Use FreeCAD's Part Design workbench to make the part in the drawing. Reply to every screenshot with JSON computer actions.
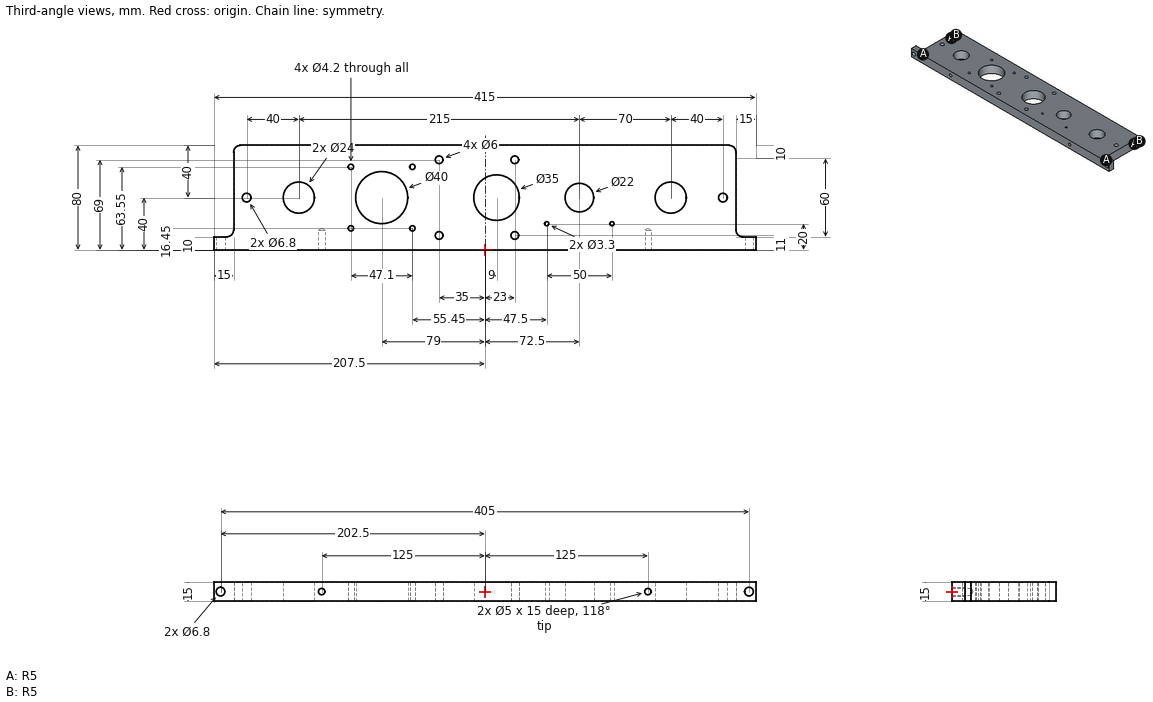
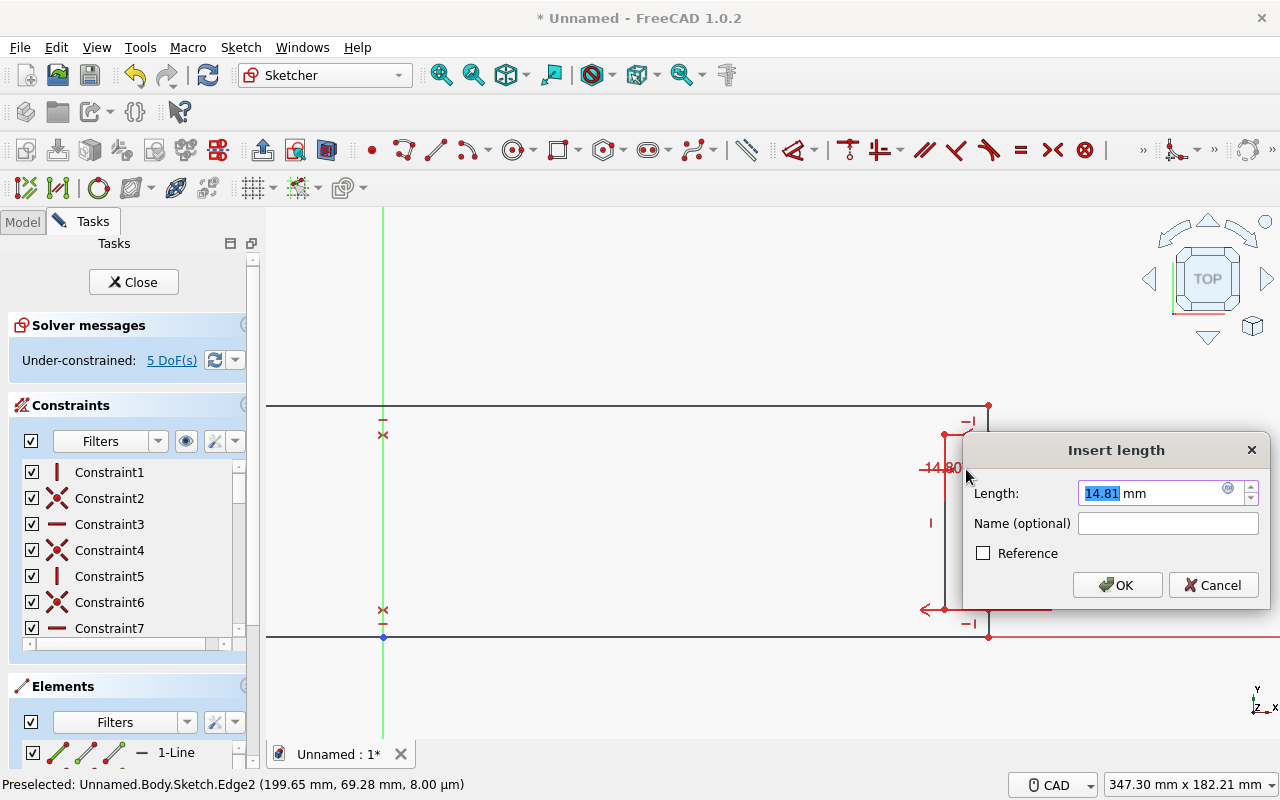
{"action": "type", "text": "15"}
{"action": "key", "text": "Return"}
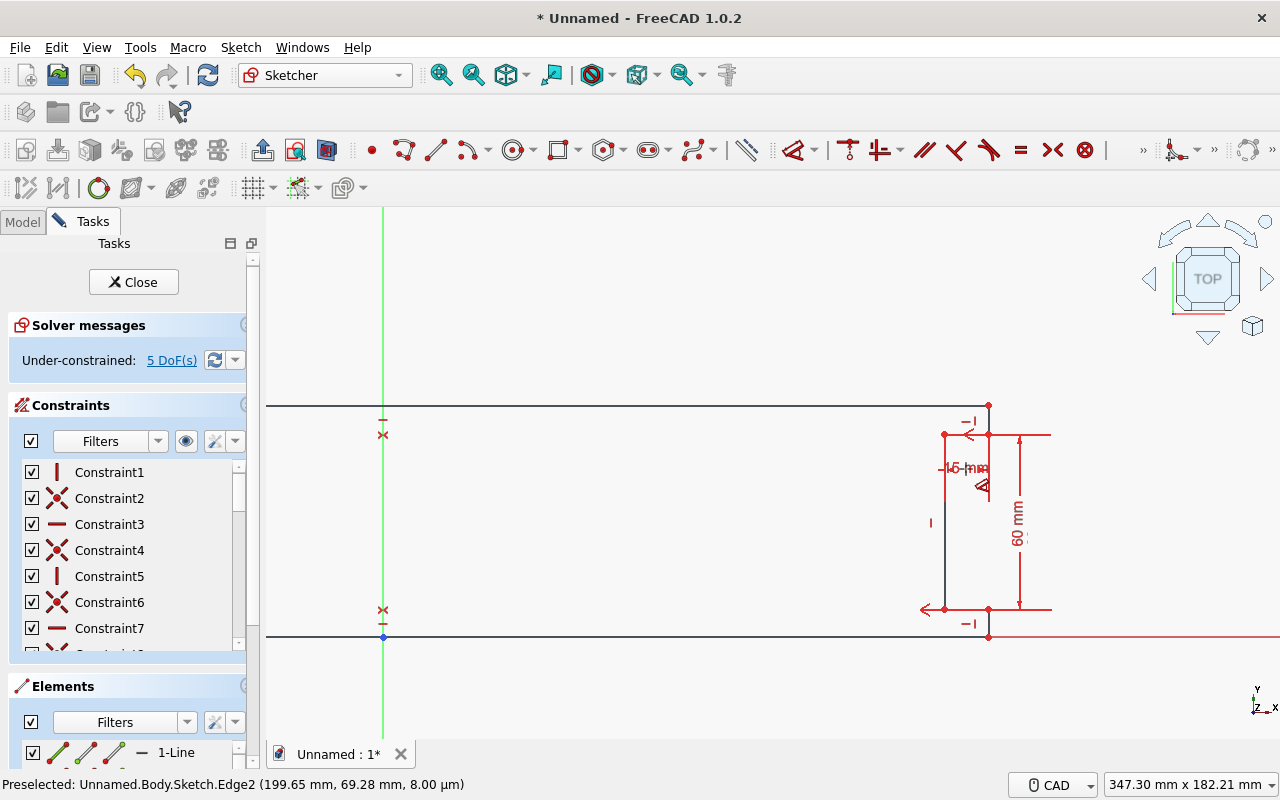
{"action": "scroll", "coordinate": [989, 423], "scroll_direction": "up", "scroll_amount": 2}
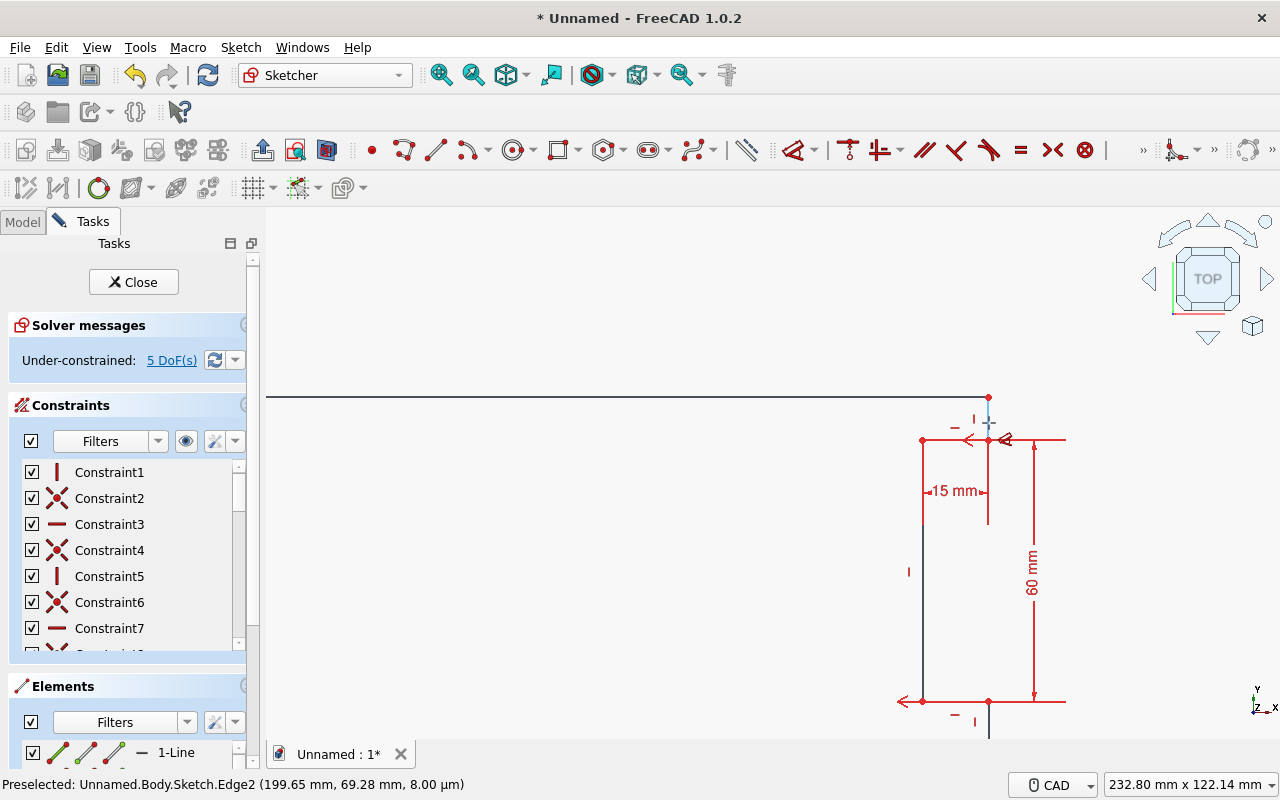
{"action": "left_click", "coordinate": [988, 423]}
{"action": "left_click", "coordinate": [1022, 419]}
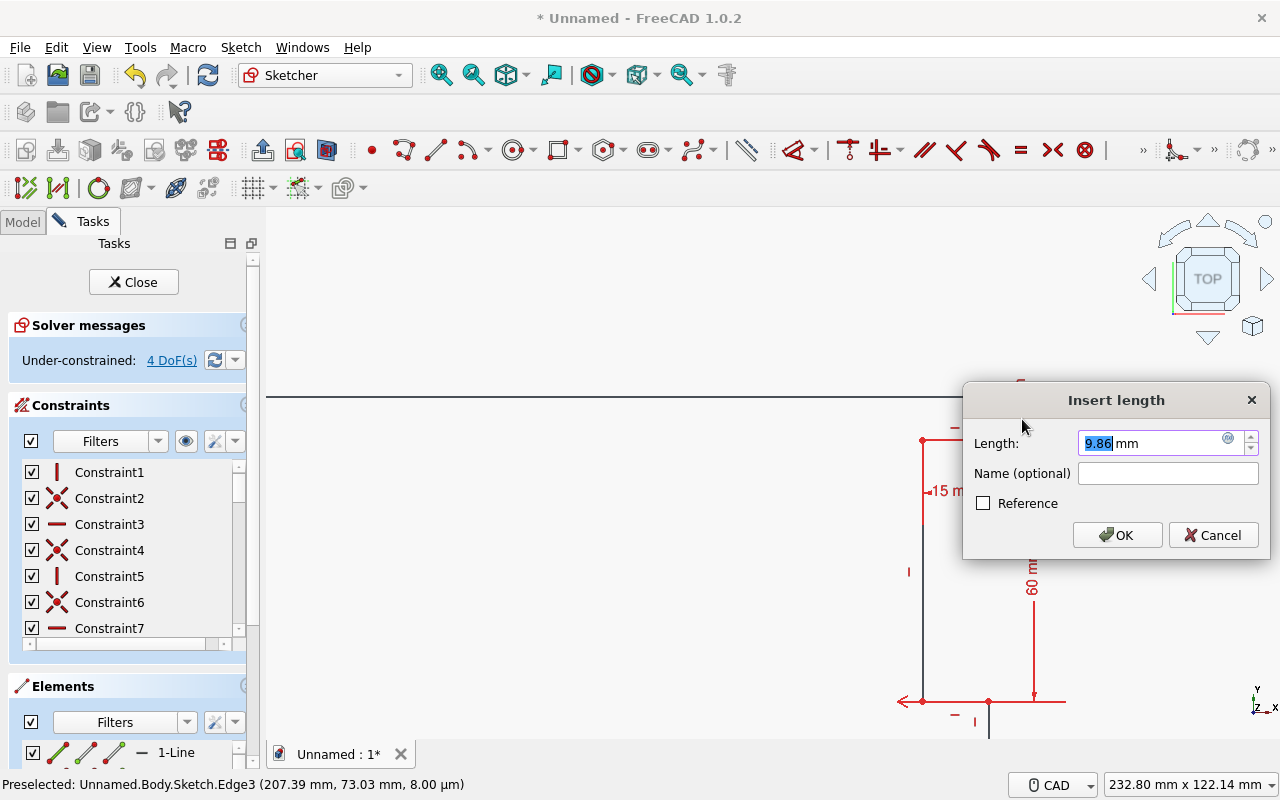
{"action": "type", "text": "10"}
{"action": "key", "text": "Return"}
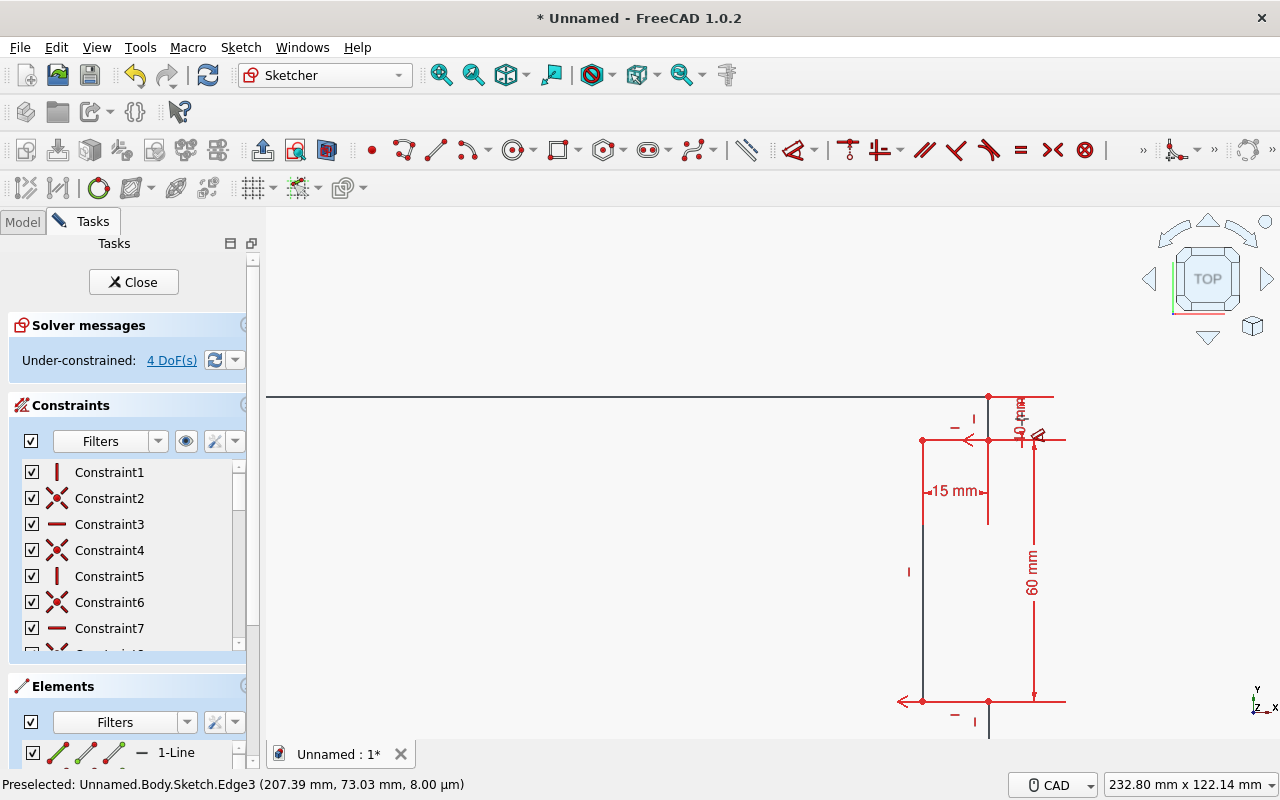
{"action": "scroll", "coordinate": [972, 432], "scroll_direction": "down", "scroll_amount": 6}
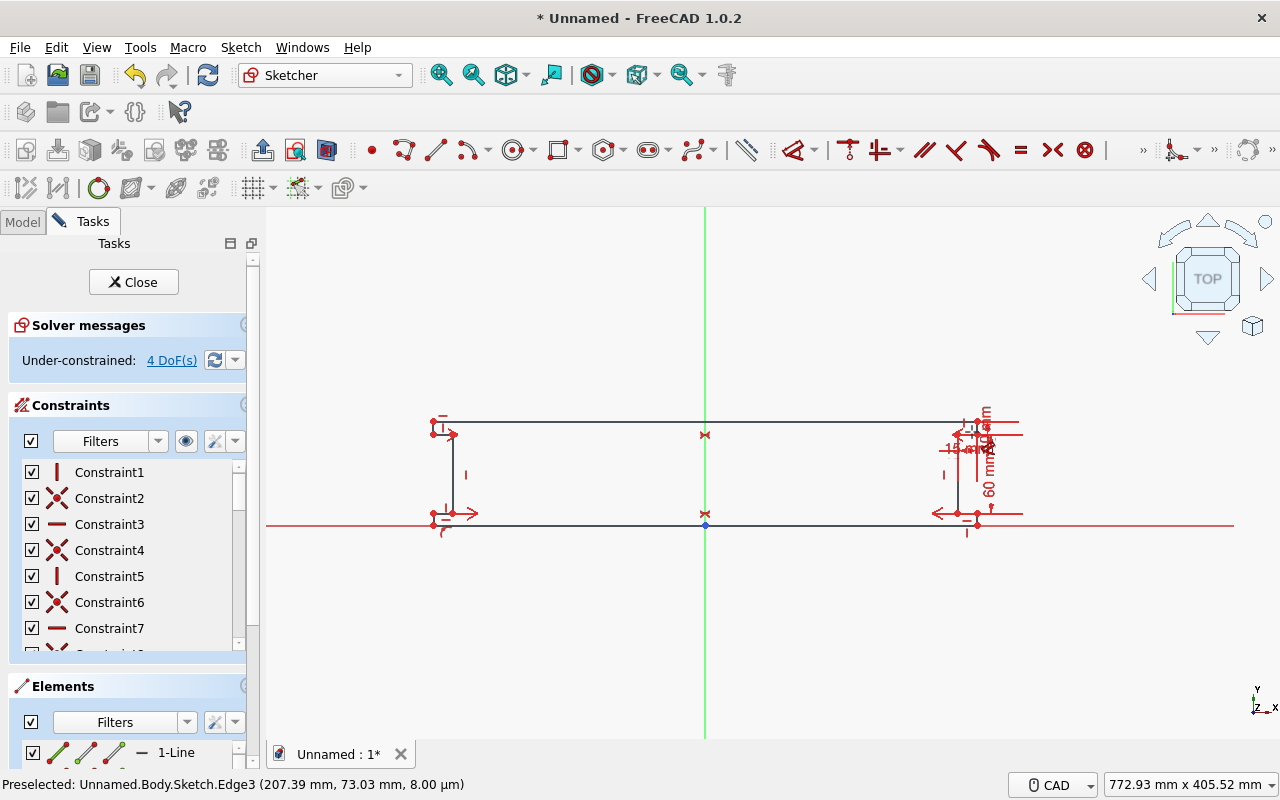
{"action": "scroll", "coordinate": [447, 514], "scroll_direction": "up", "scroll_amount": 5}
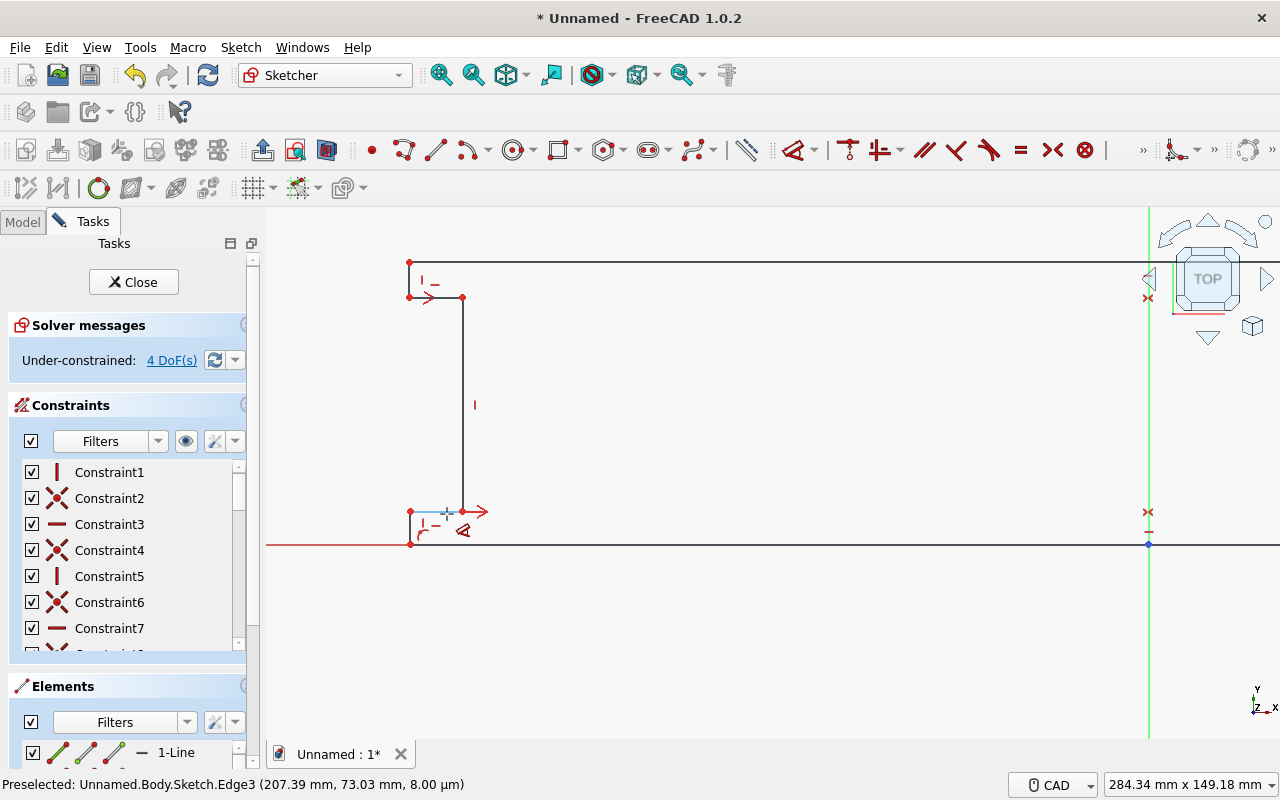
{"action": "left_click", "coordinate": [447, 512]}
{"action": "left_click", "coordinate": [436, 478]}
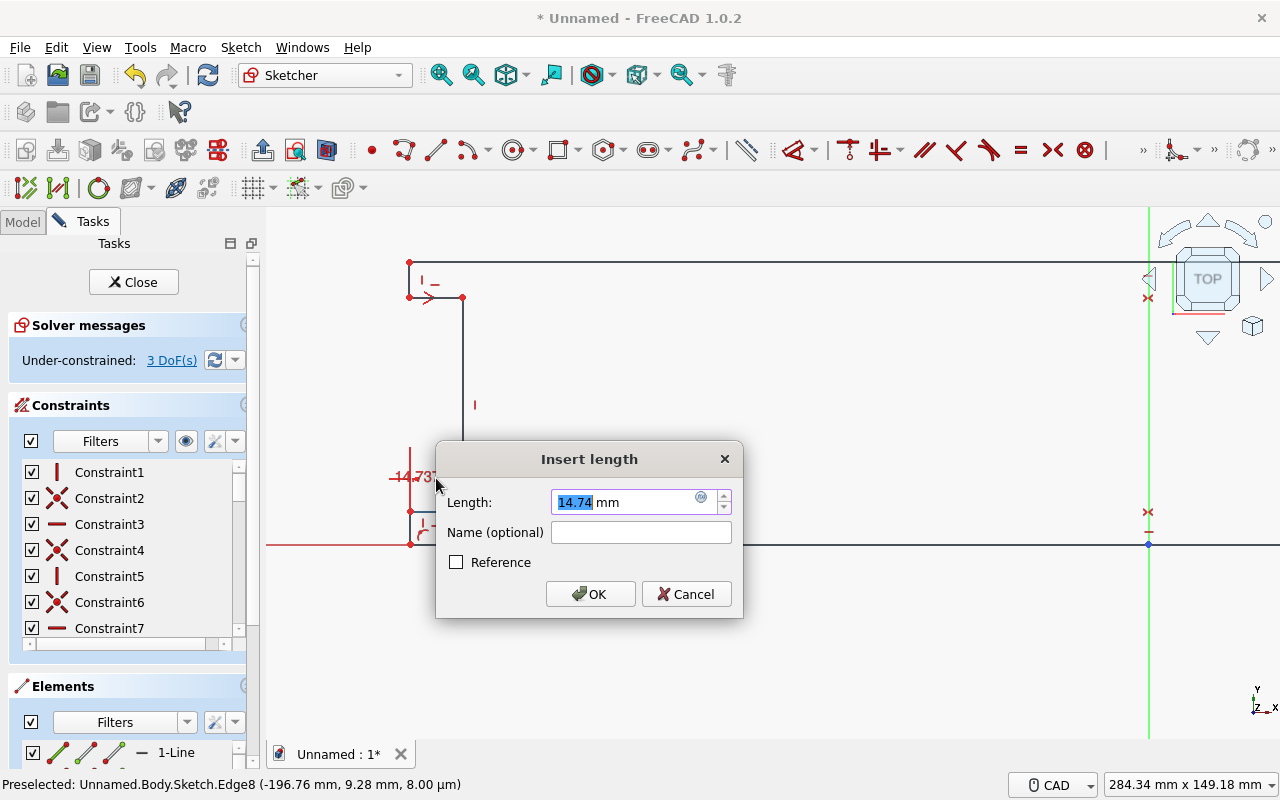
{"action": "type", "text": "15"}
{"action": "key", "text": "Return"}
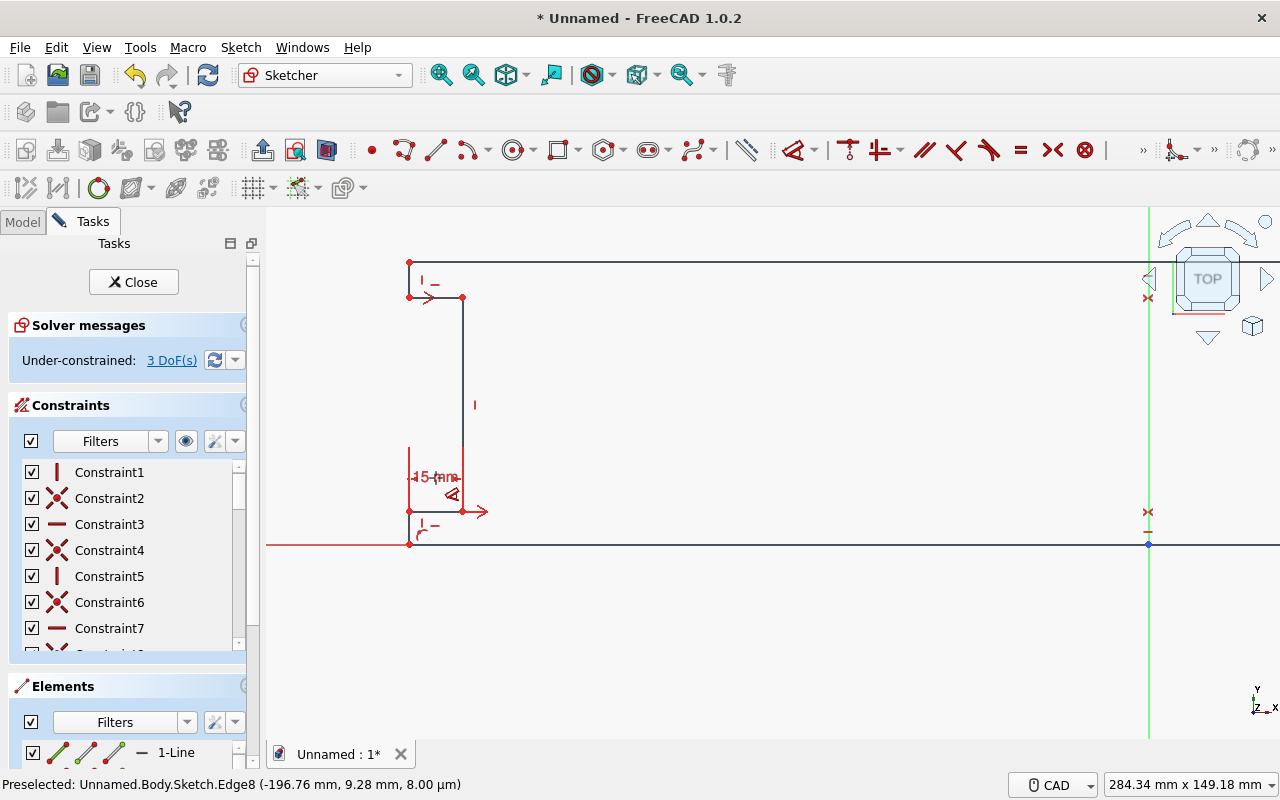
{"action": "scroll", "coordinate": [409, 522], "scroll_direction": "up", "scroll_amount": 2}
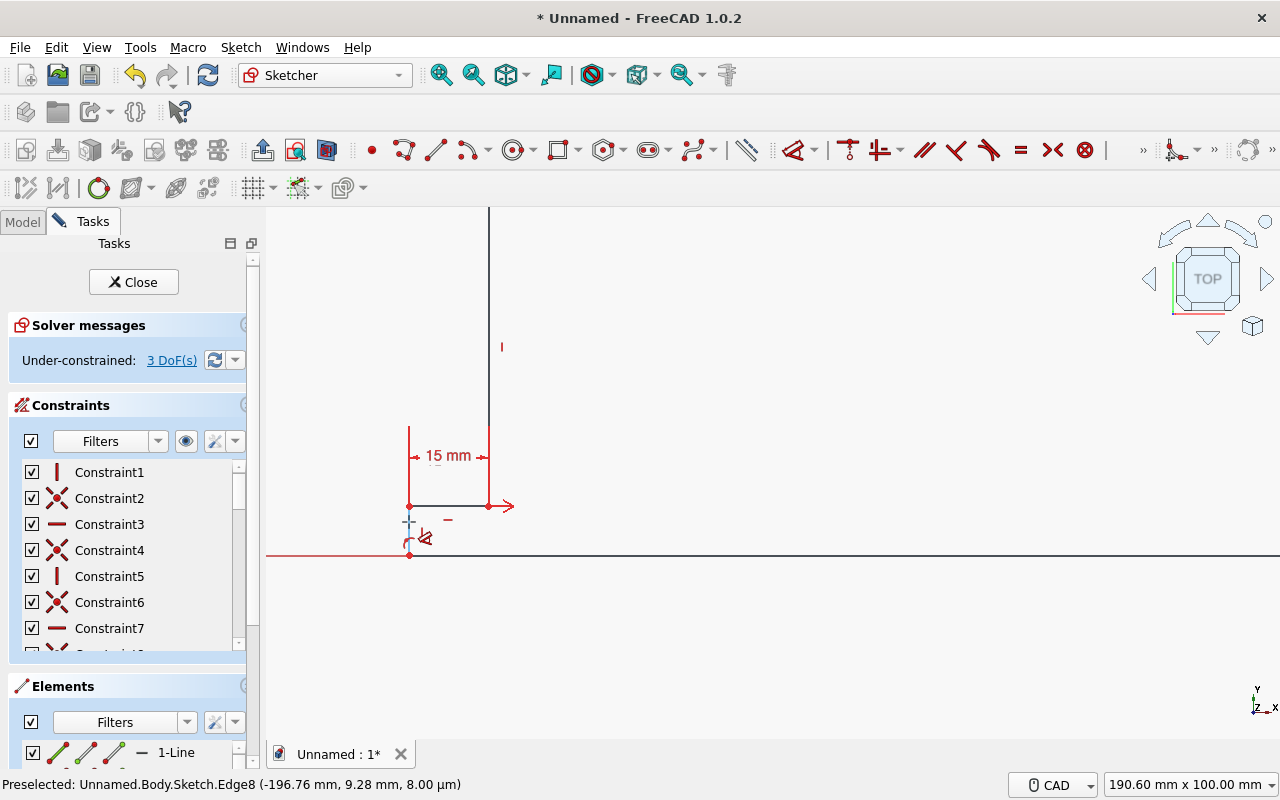
{"action": "left_click", "coordinate": [409, 521]}
{"action": "left_click", "coordinate": [375, 531]}